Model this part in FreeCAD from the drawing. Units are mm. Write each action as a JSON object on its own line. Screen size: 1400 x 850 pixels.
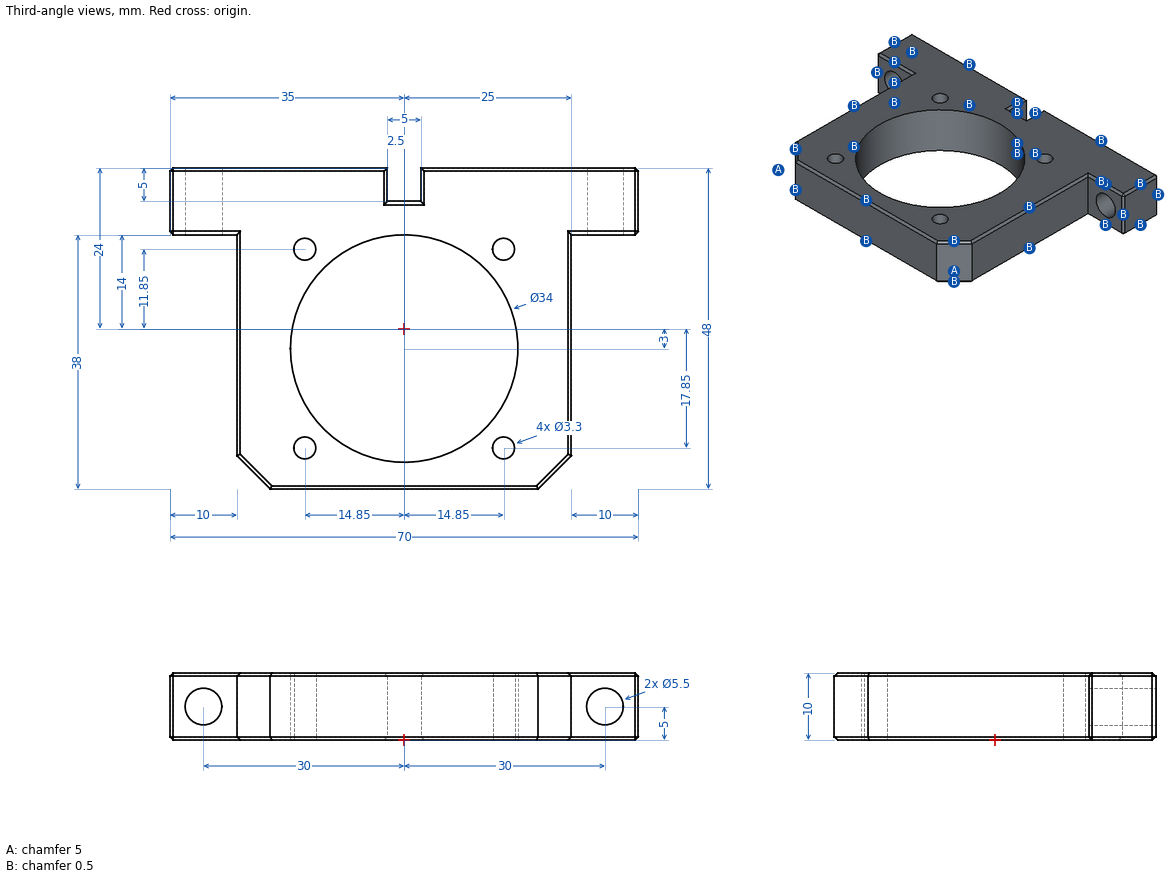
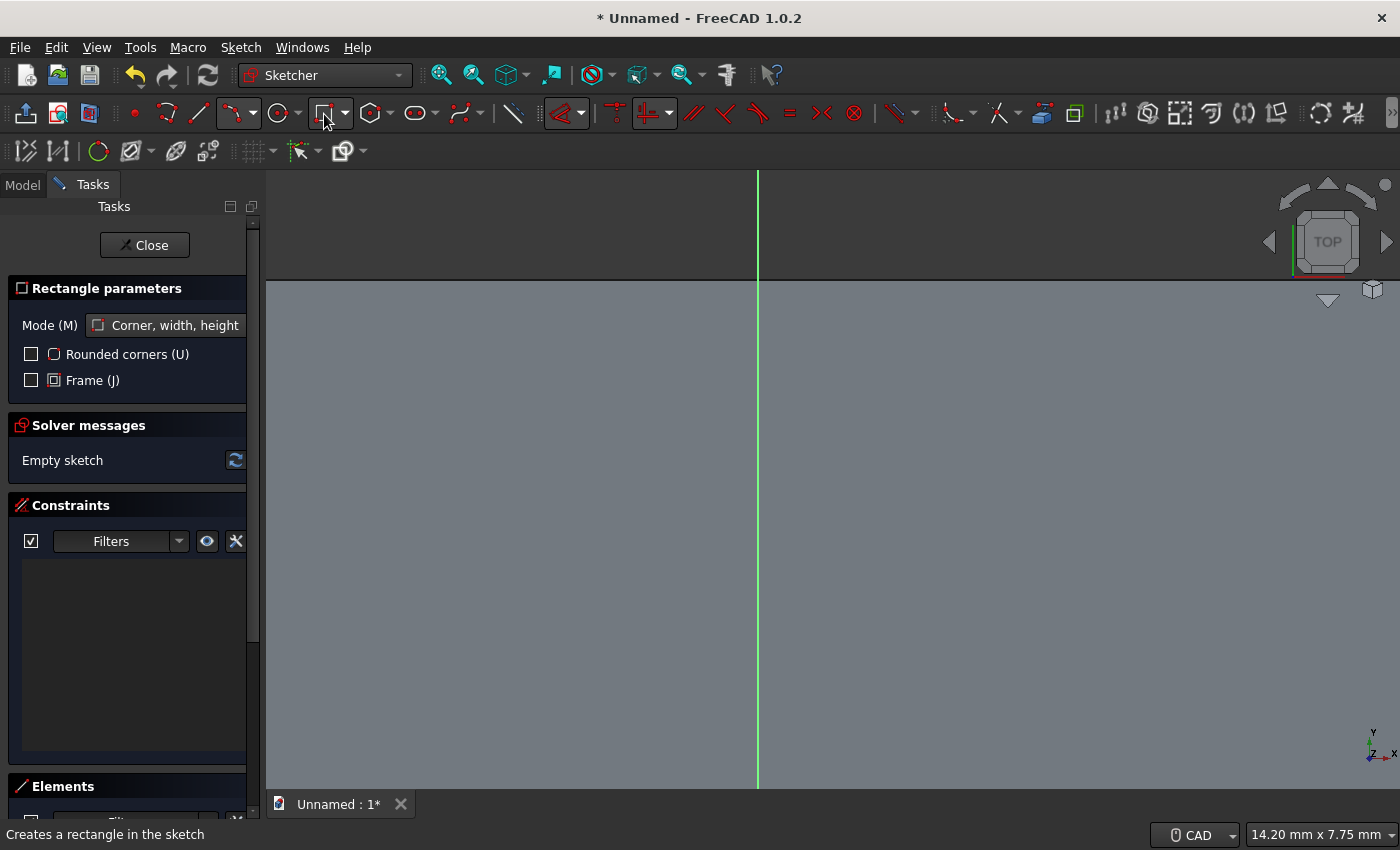
{"action": "left_click", "coordinate": [558, 280]}
{"action": "left_click", "coordinate": [957, 679]}
{"action": "key", "text": "Escape"}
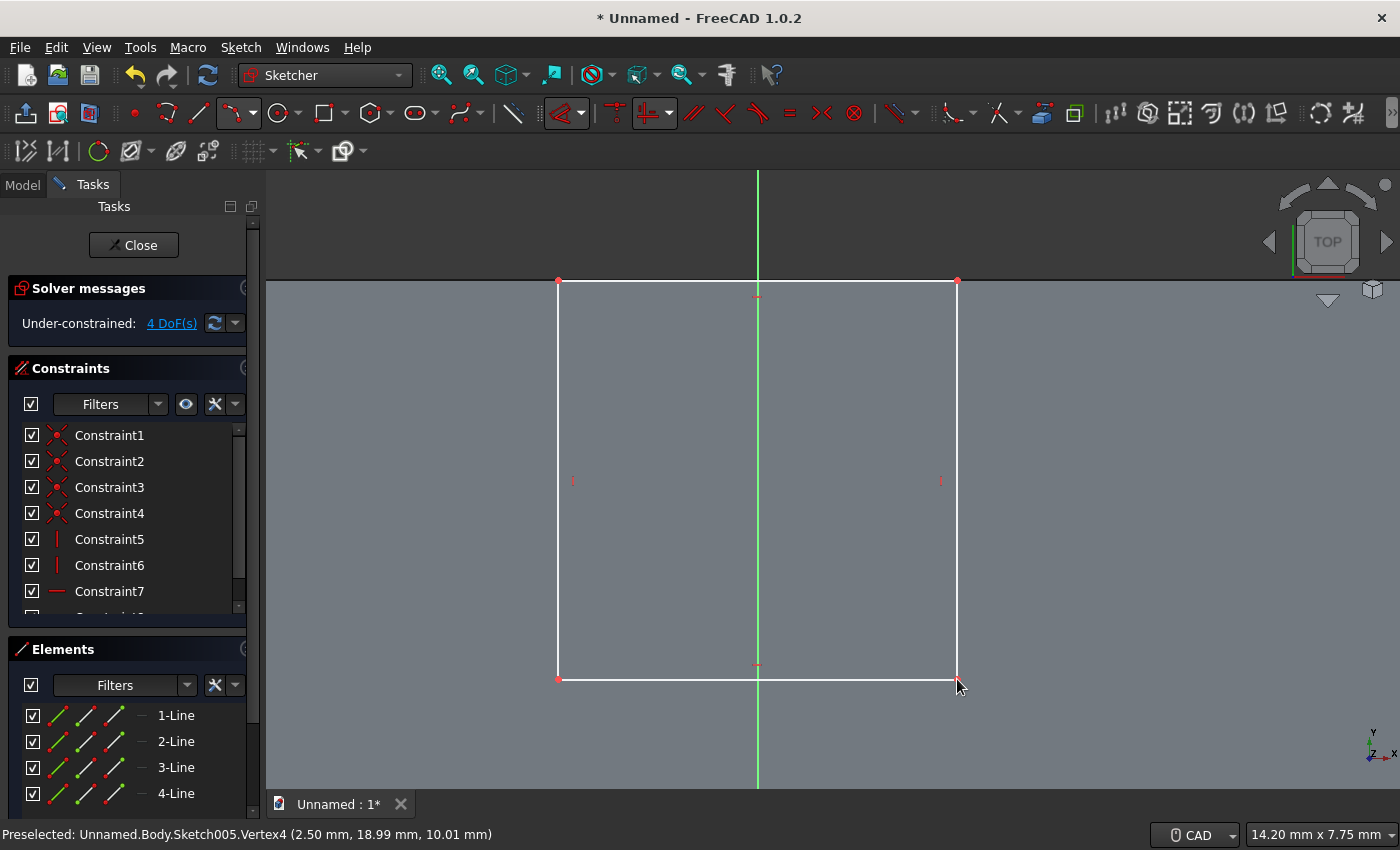
{"action": "left_click", "coordinate": [558, 401]}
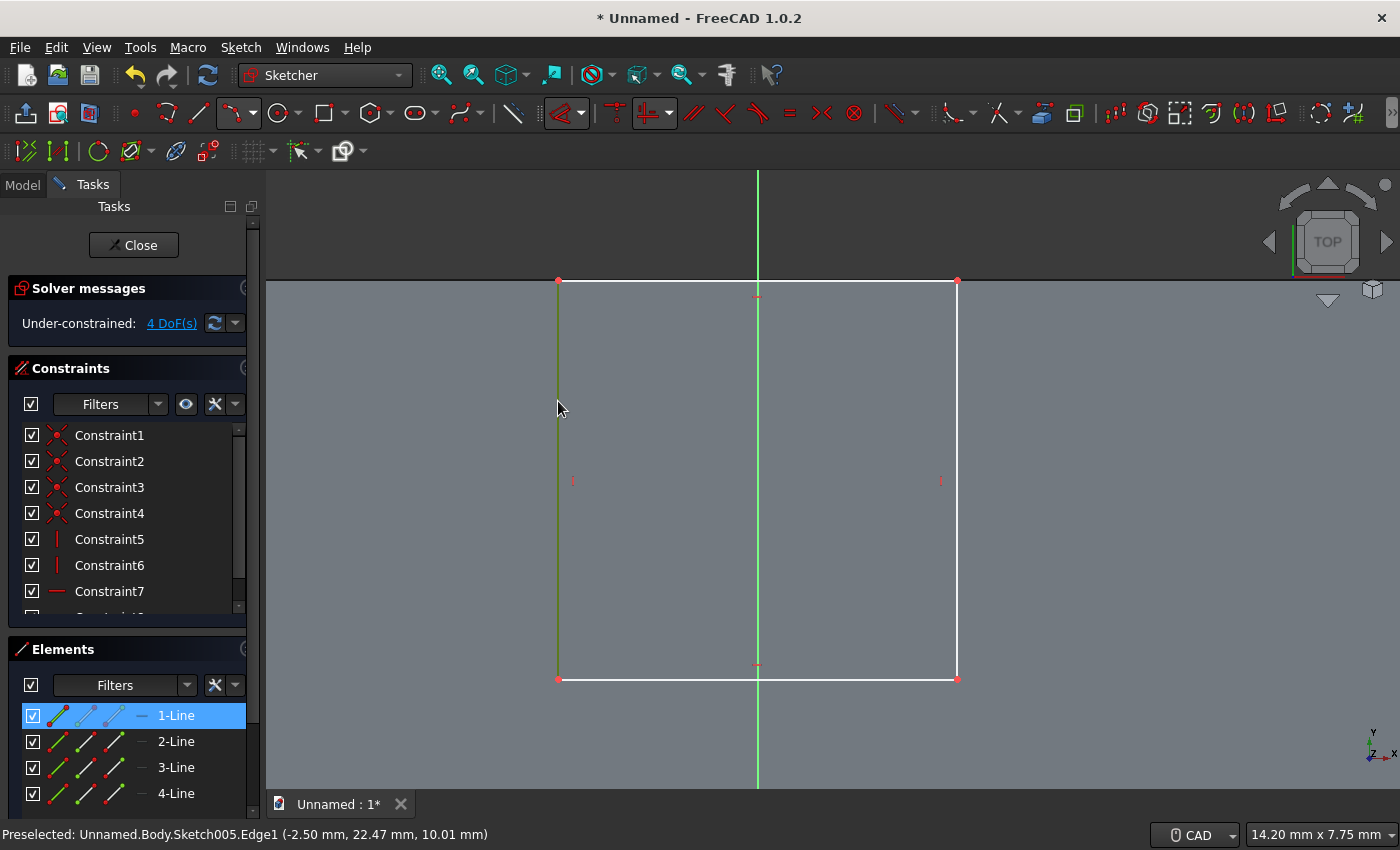
{"action": "left_click", "coordinate": [584, 114]}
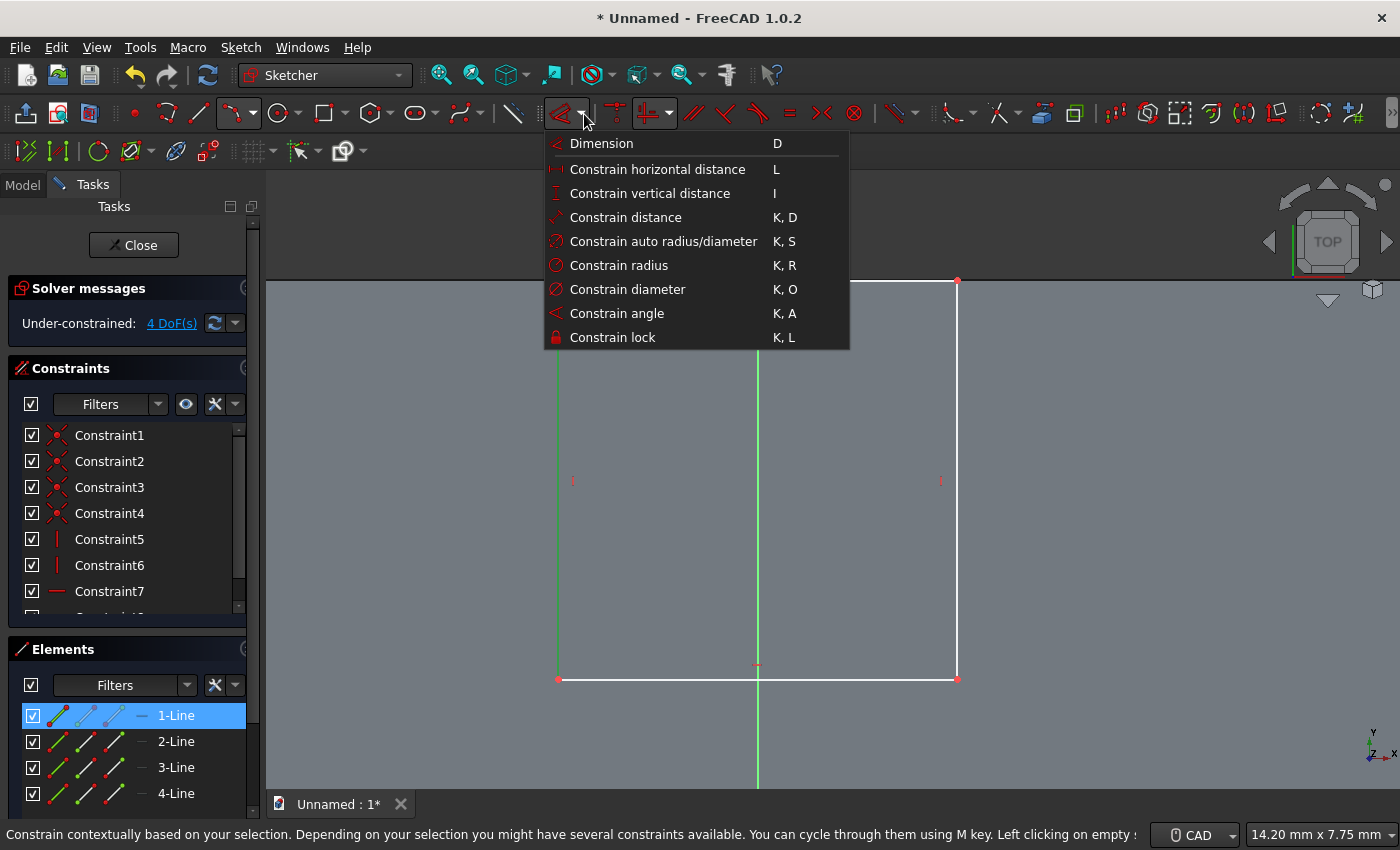
{"action": "left_click", "coordinate": [697, 193]}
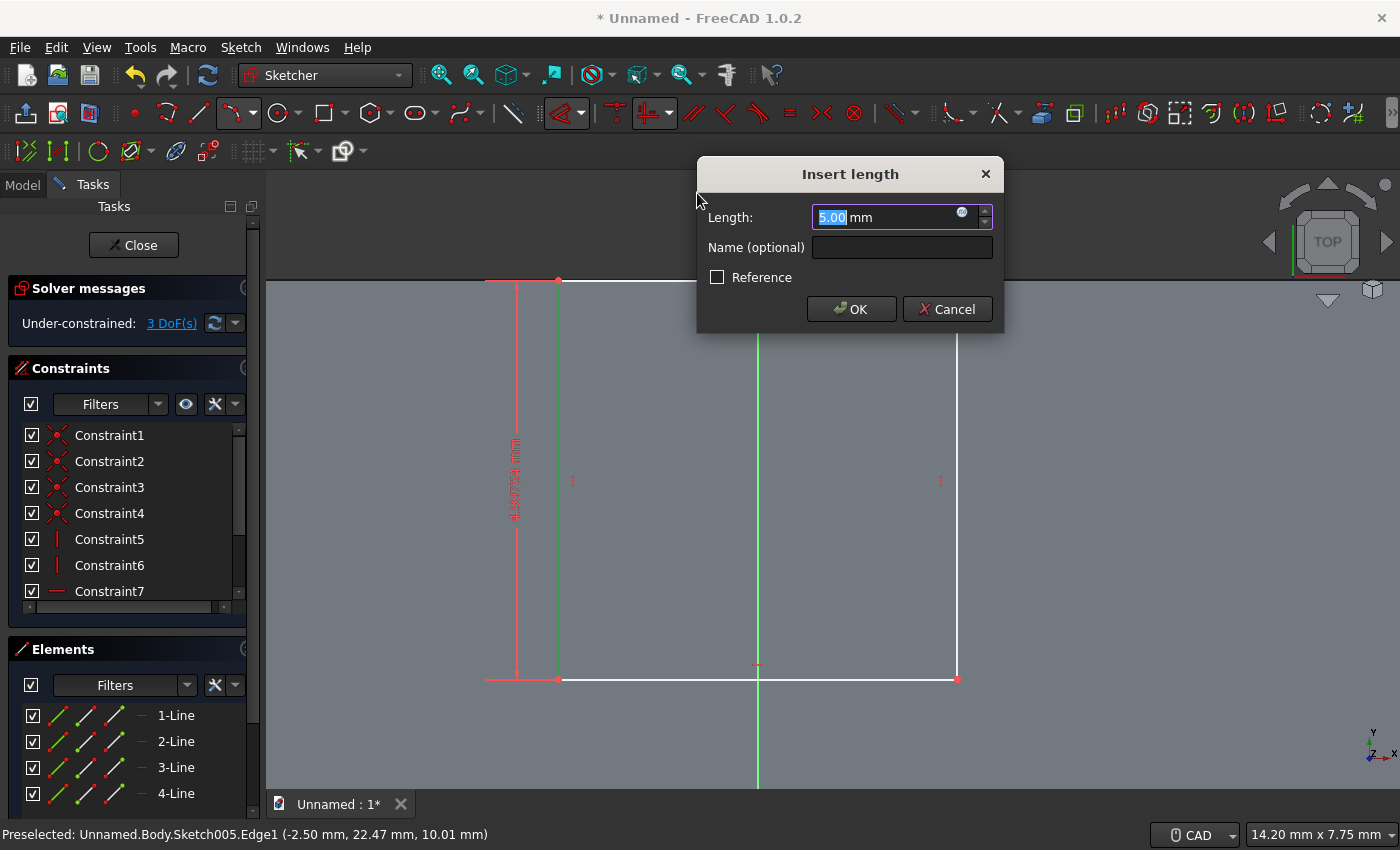
{"action": "type", "text": "5"}
{"action": "key", "text": "Return"}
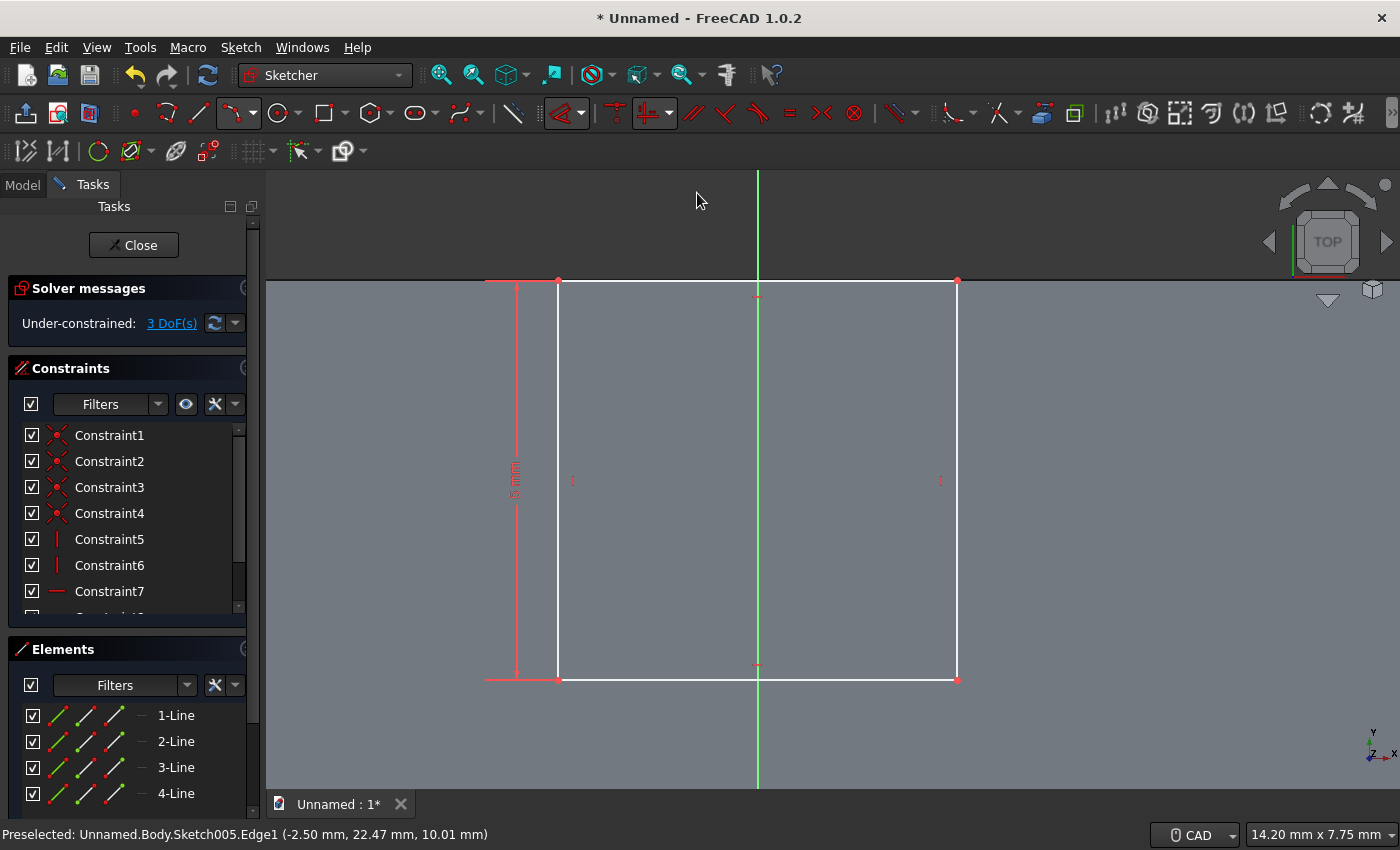
{"action": "left_click", "coordinate": [678, 680]}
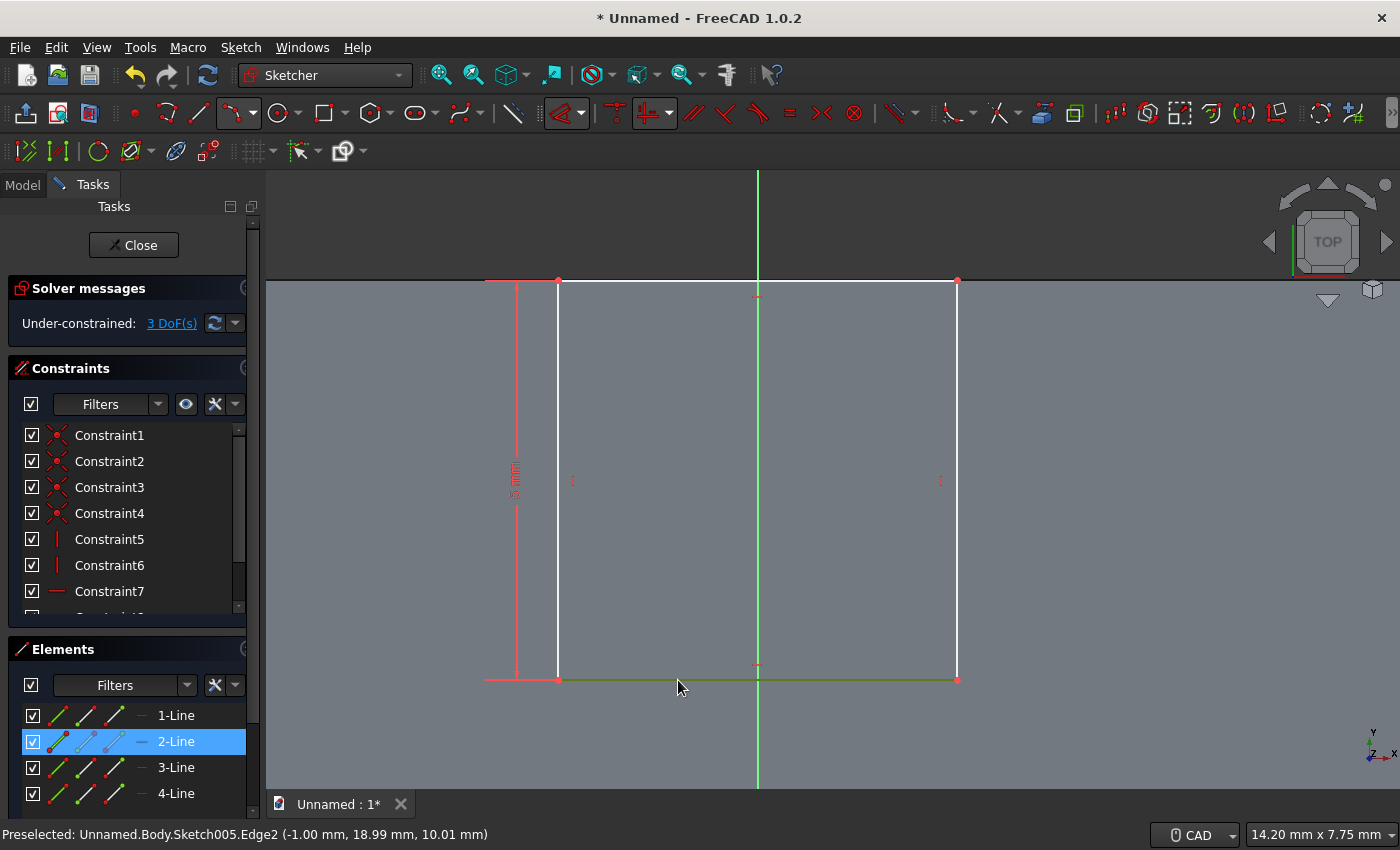
{"action": "left_click", "coordinate": [584, 114]}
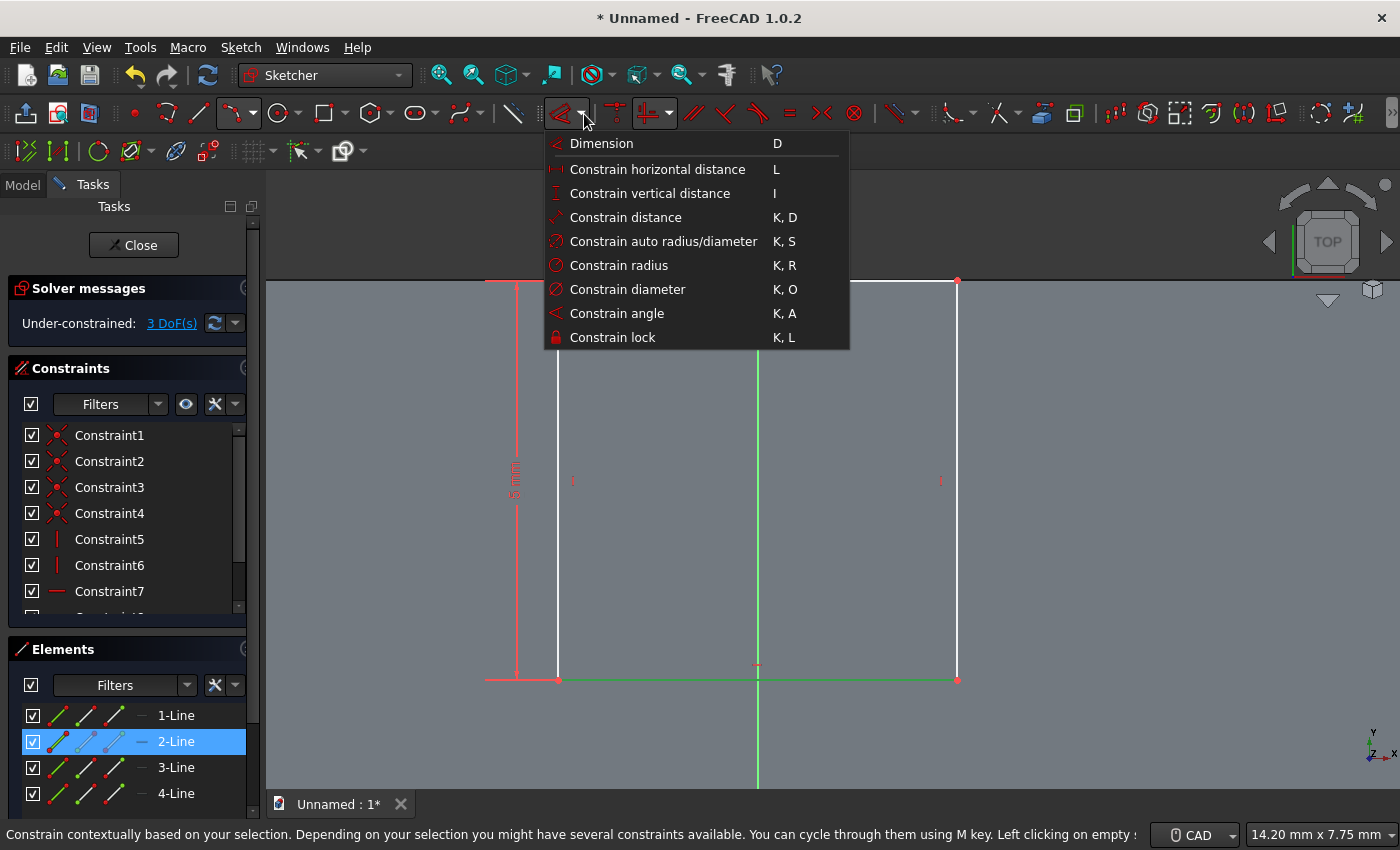
{"action": "left_click", "coordinate": [697, 169]}